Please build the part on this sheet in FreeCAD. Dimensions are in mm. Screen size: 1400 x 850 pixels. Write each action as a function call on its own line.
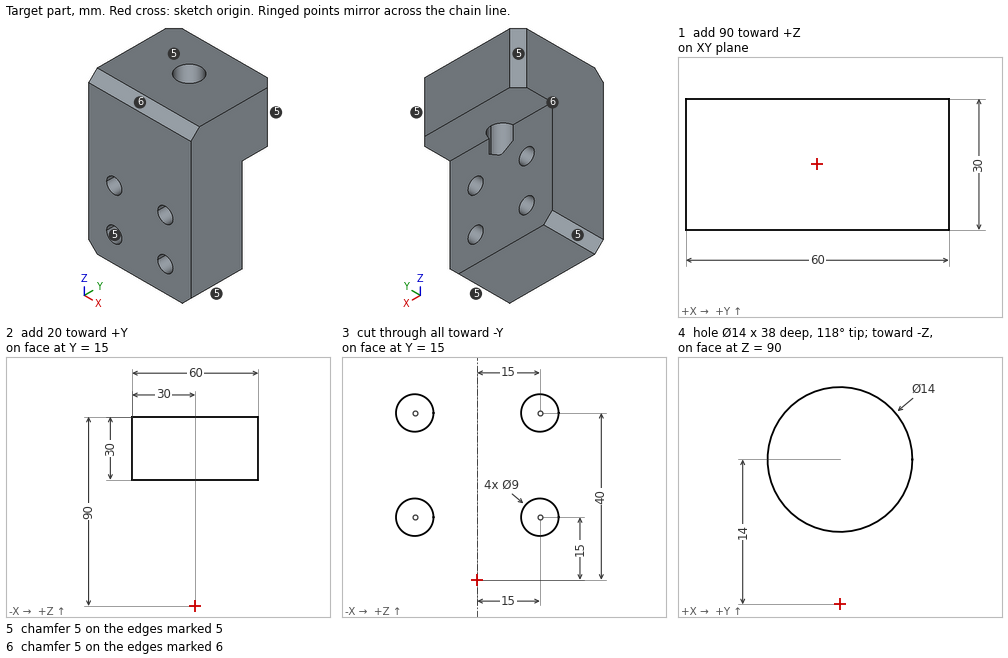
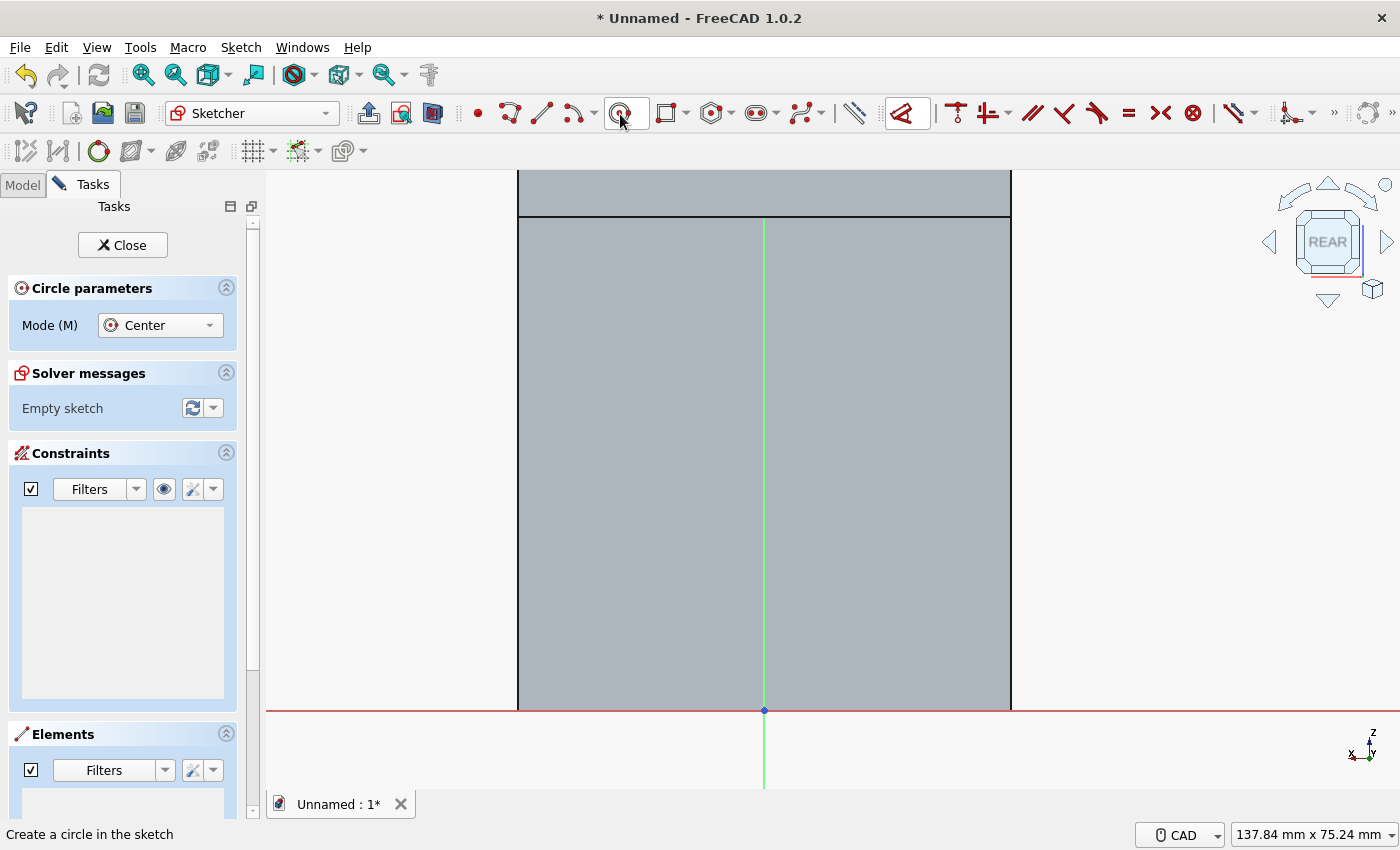
click(888, 587)
click(914, 561)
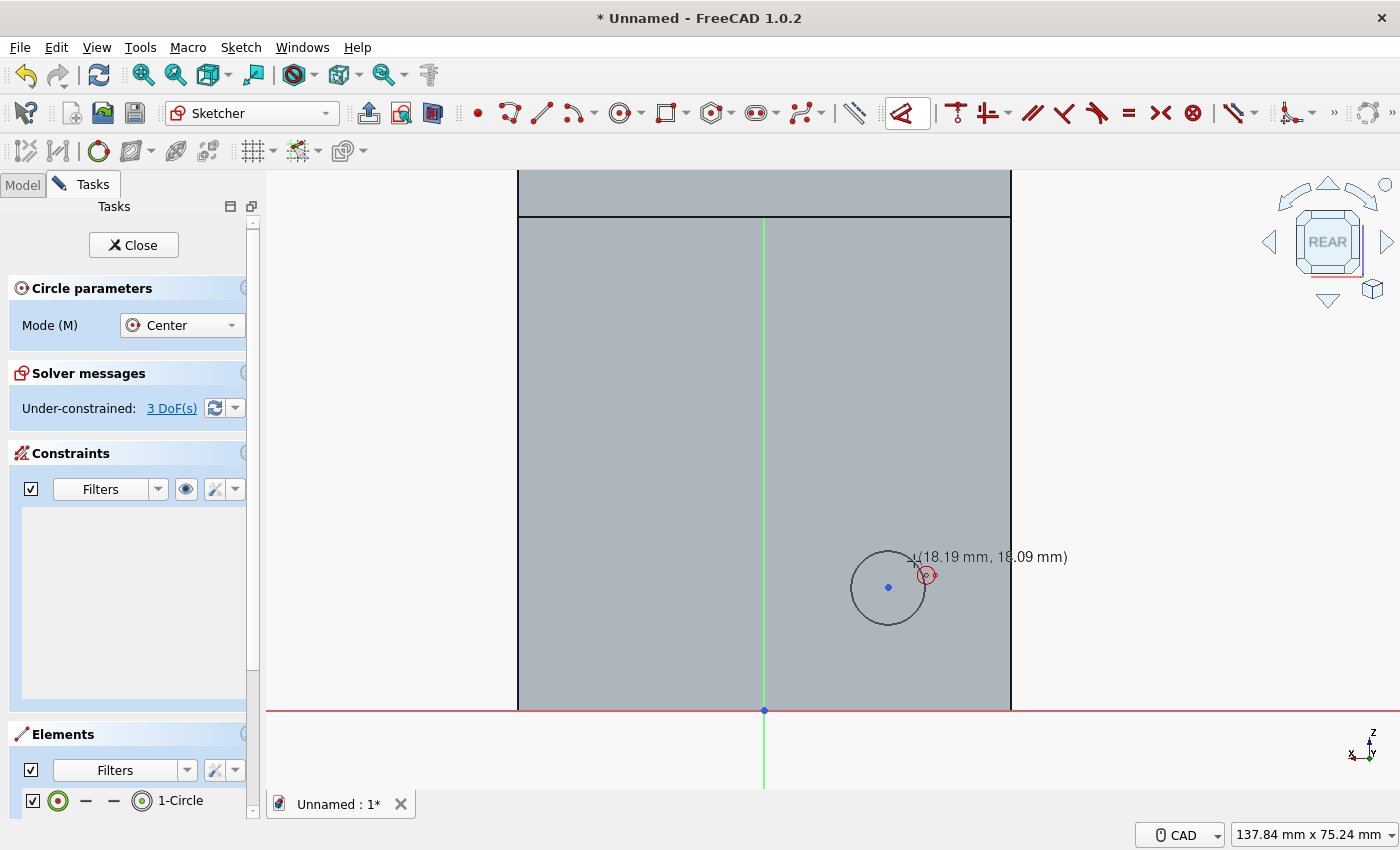
click(641, 587)
click(667, 561)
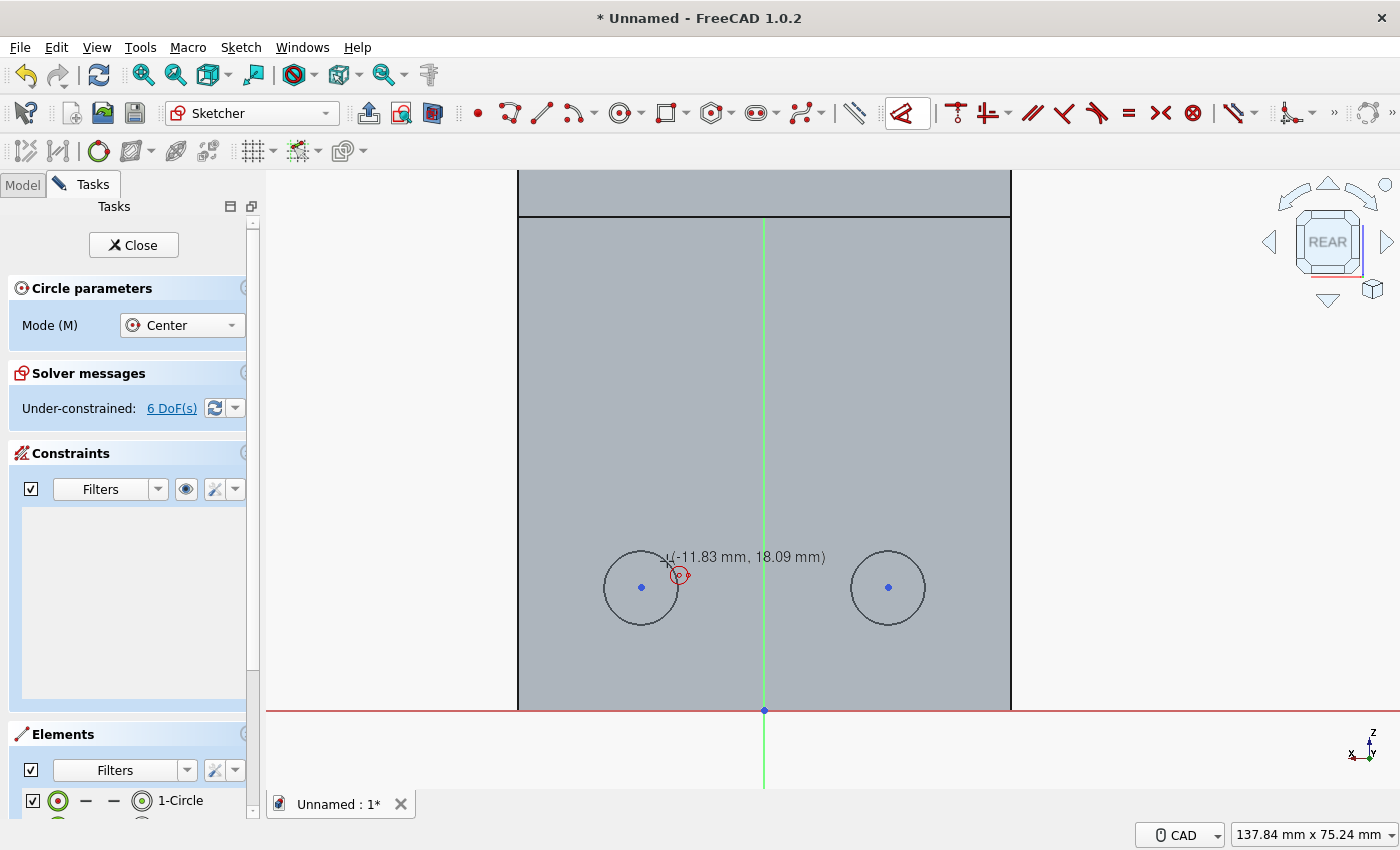
click(888, 382)
click(914, 356)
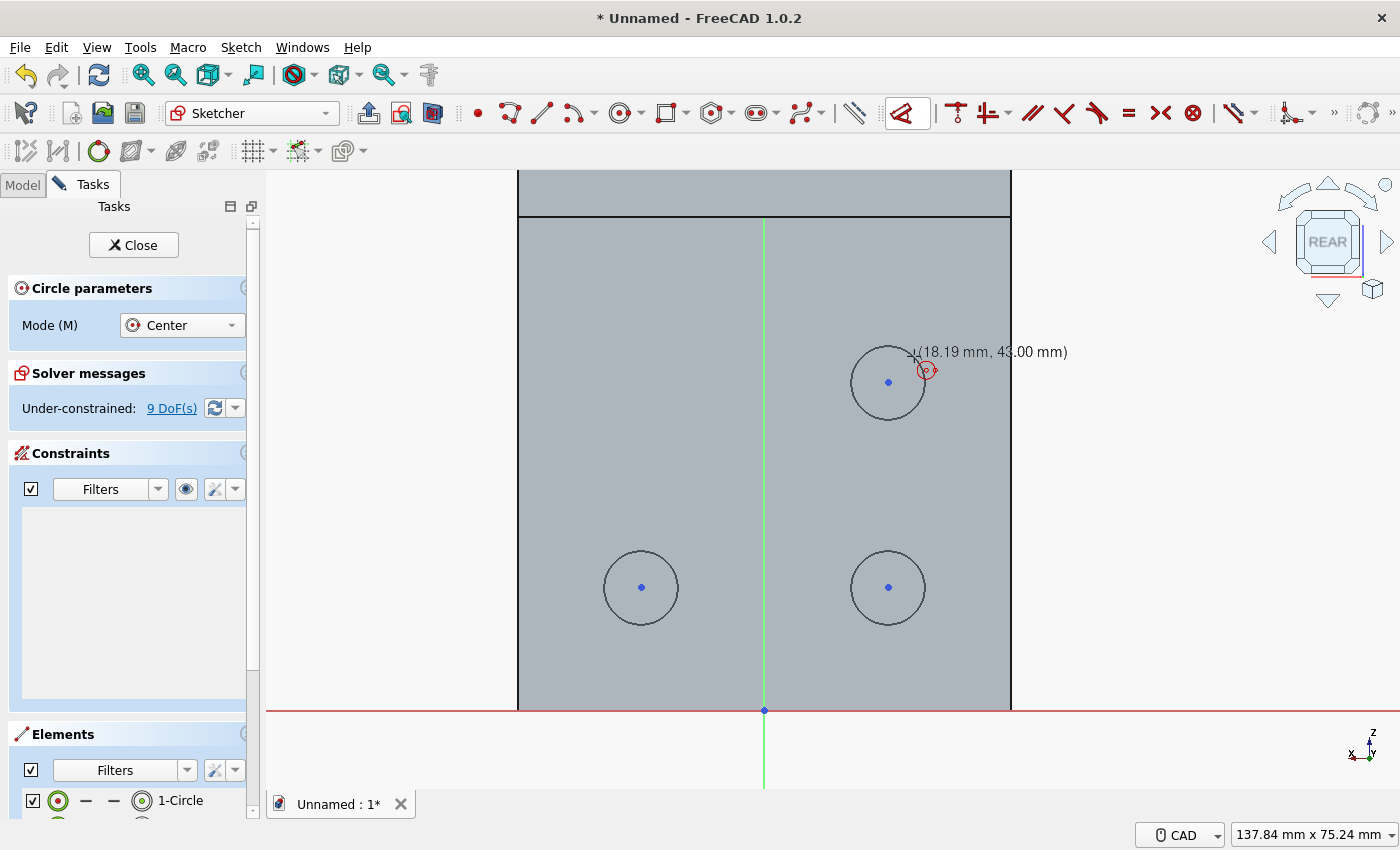
click(641, 382)
click(667, 356)
key(Escape)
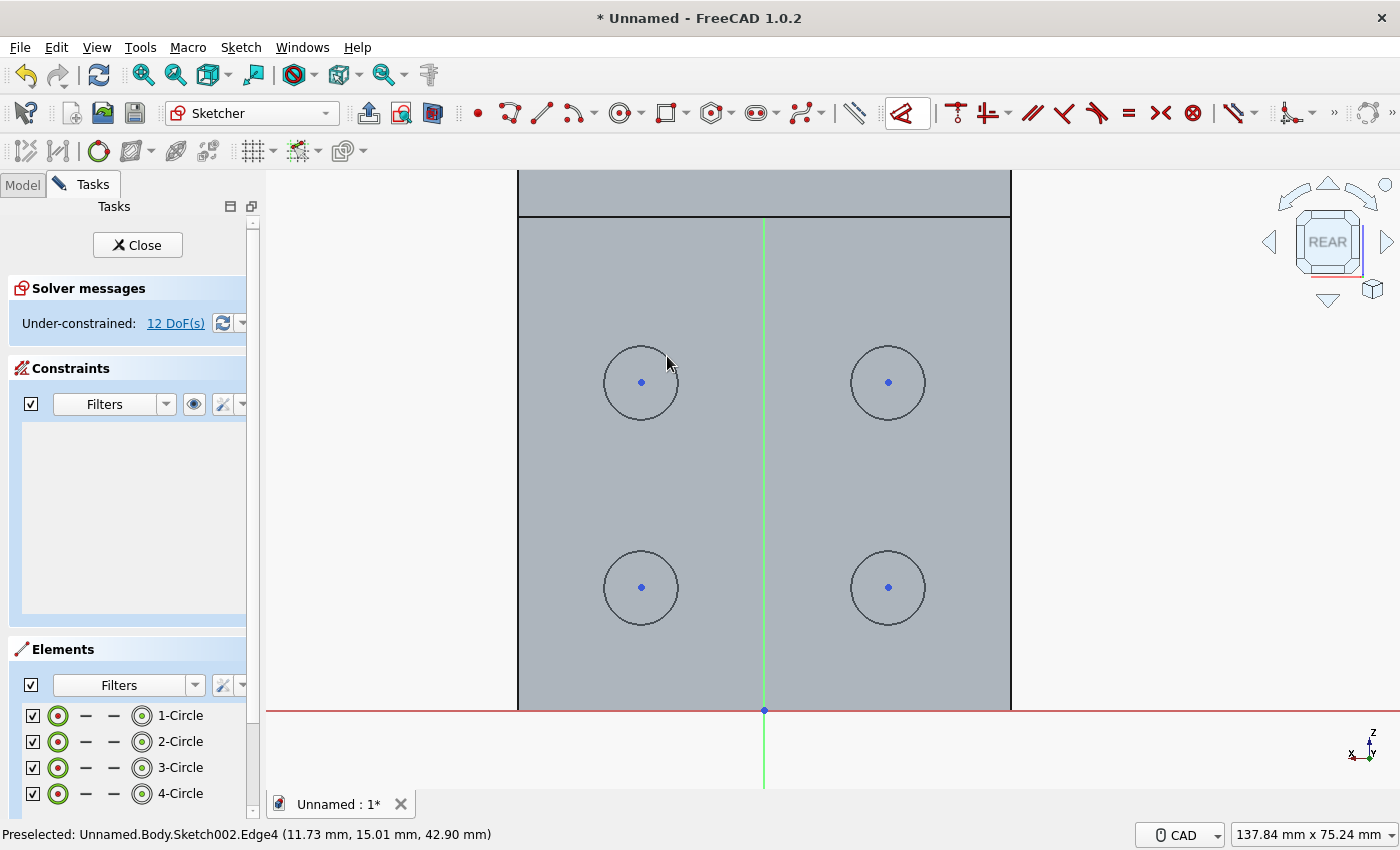
click(914, 562)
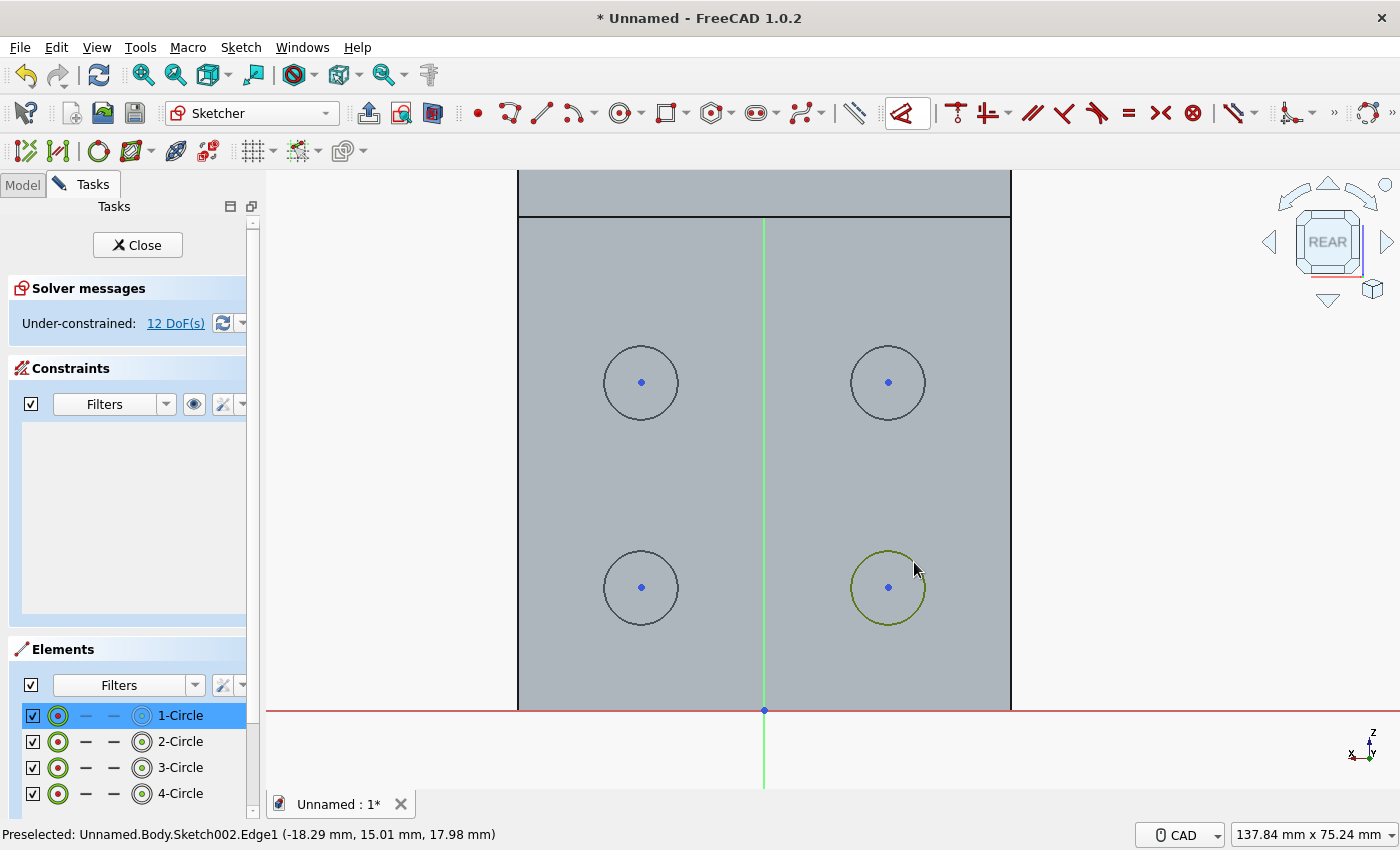
click(667, 562)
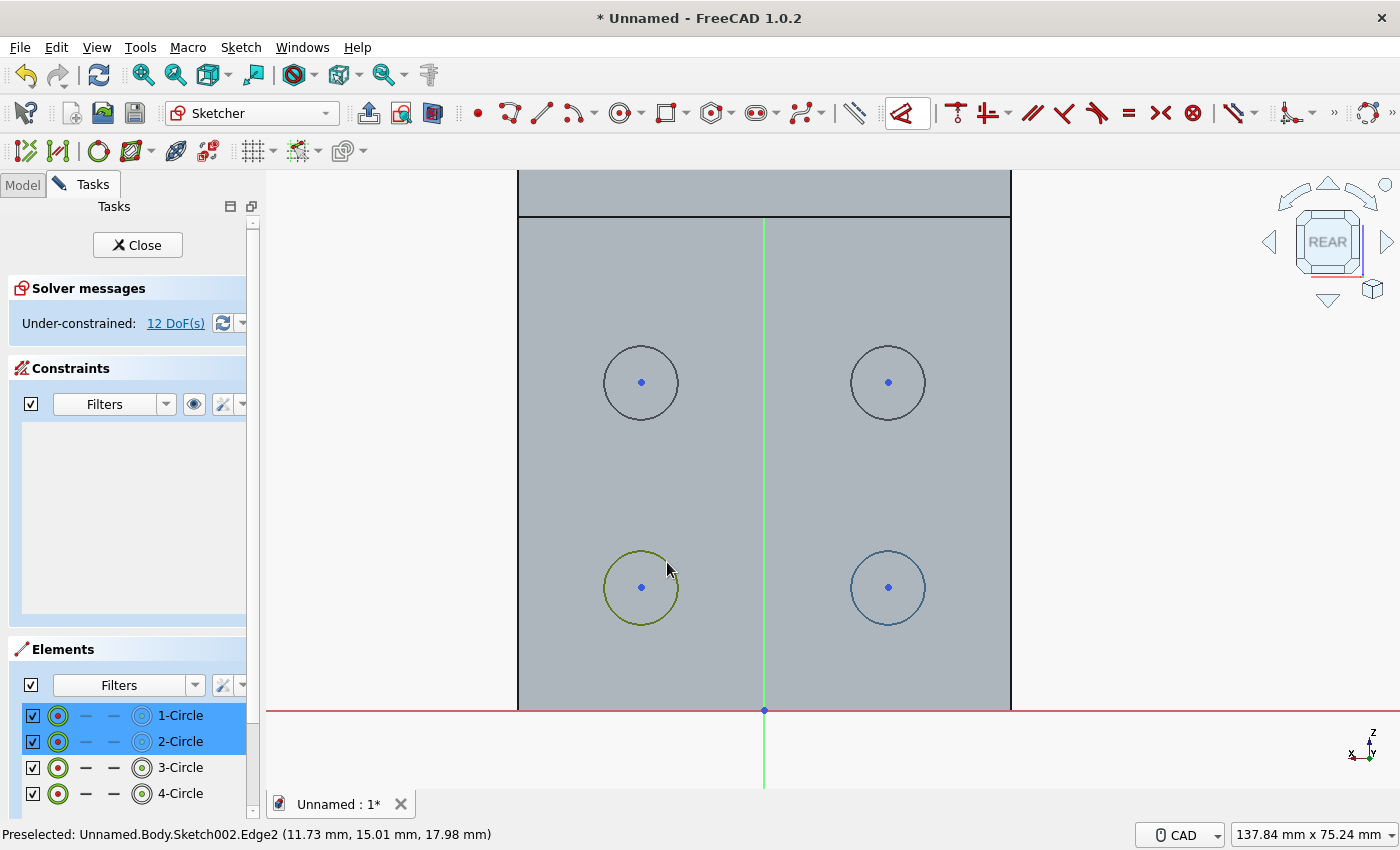
click(914, 357)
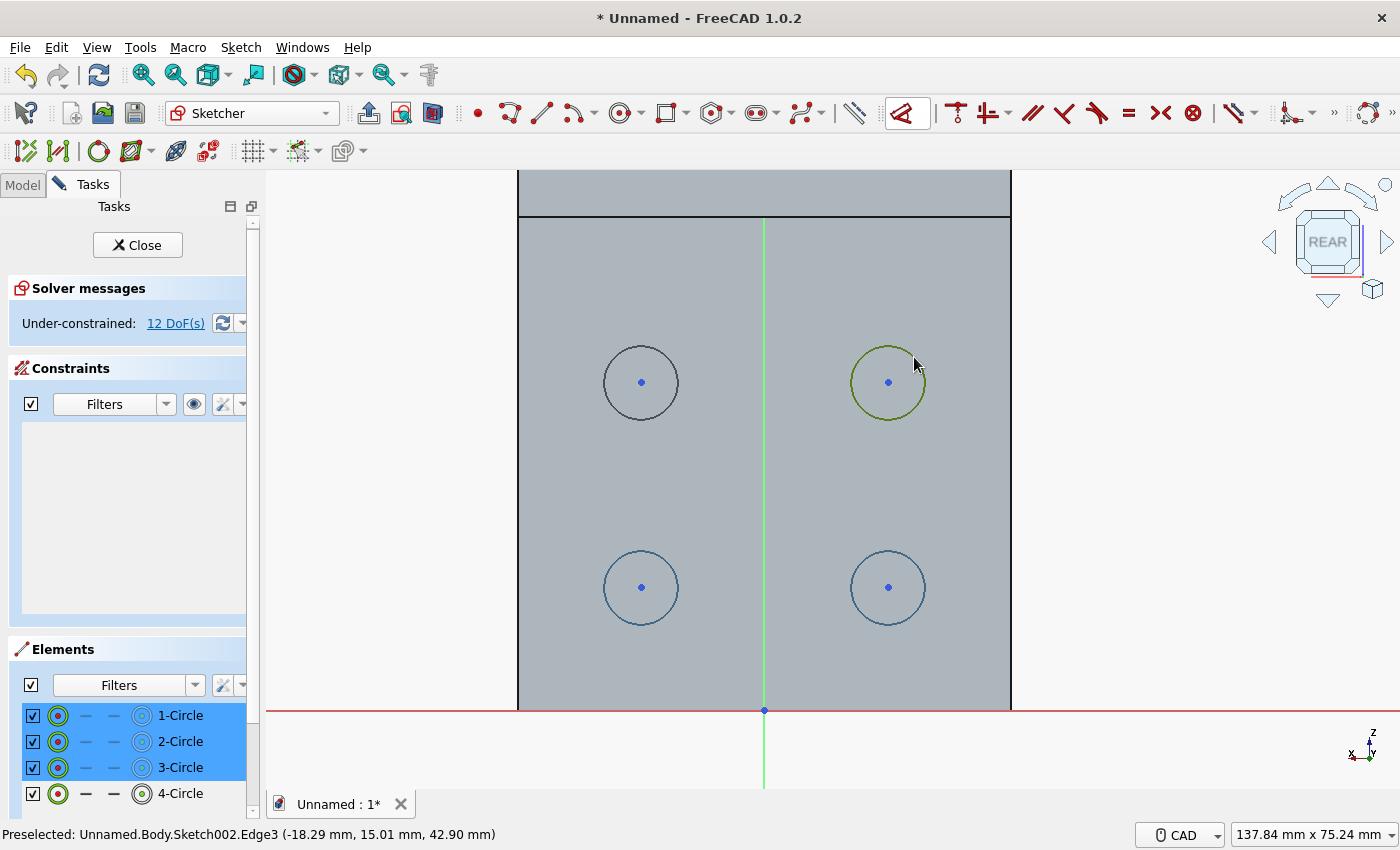
click(667, 357)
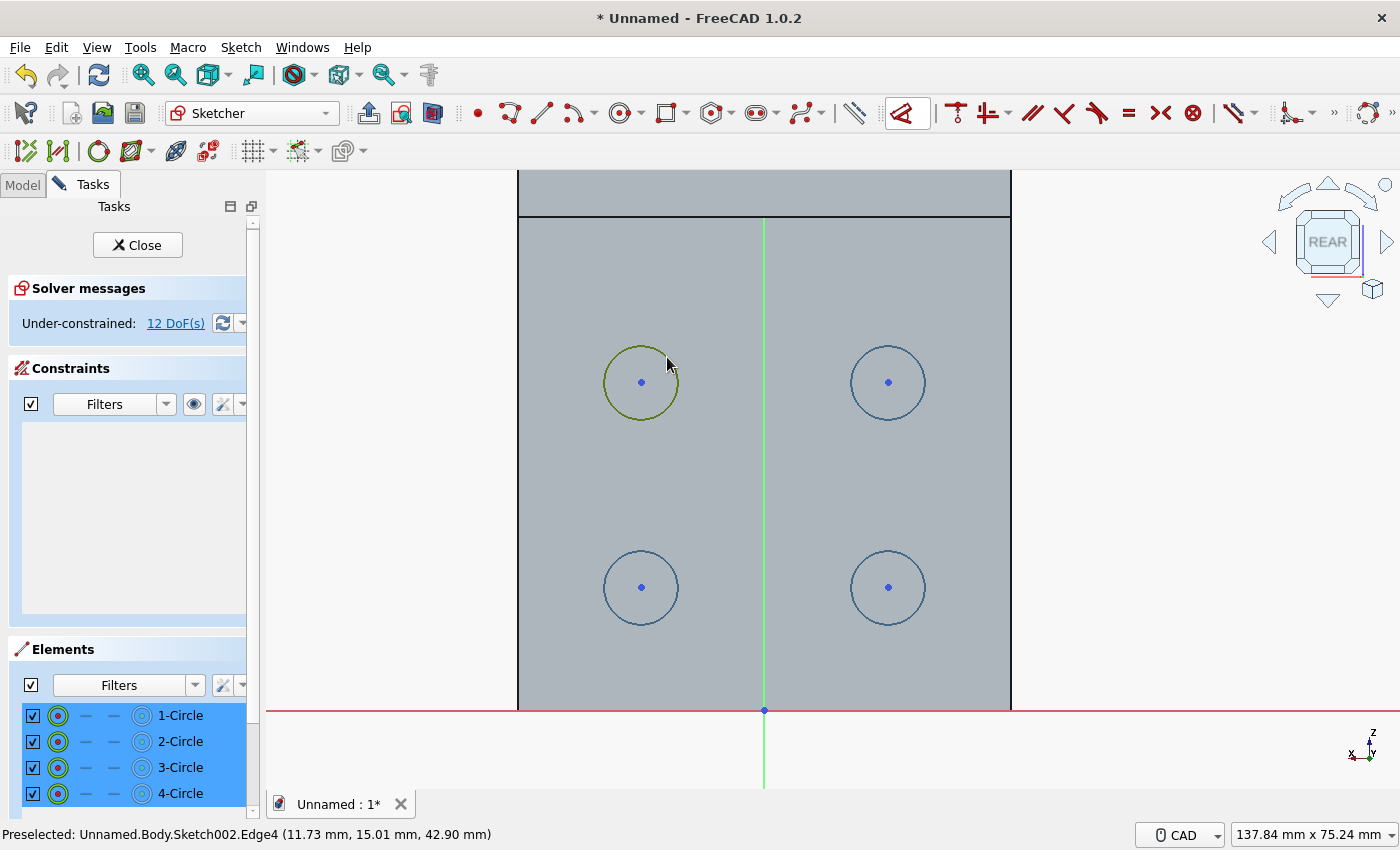
click(1130, 114)